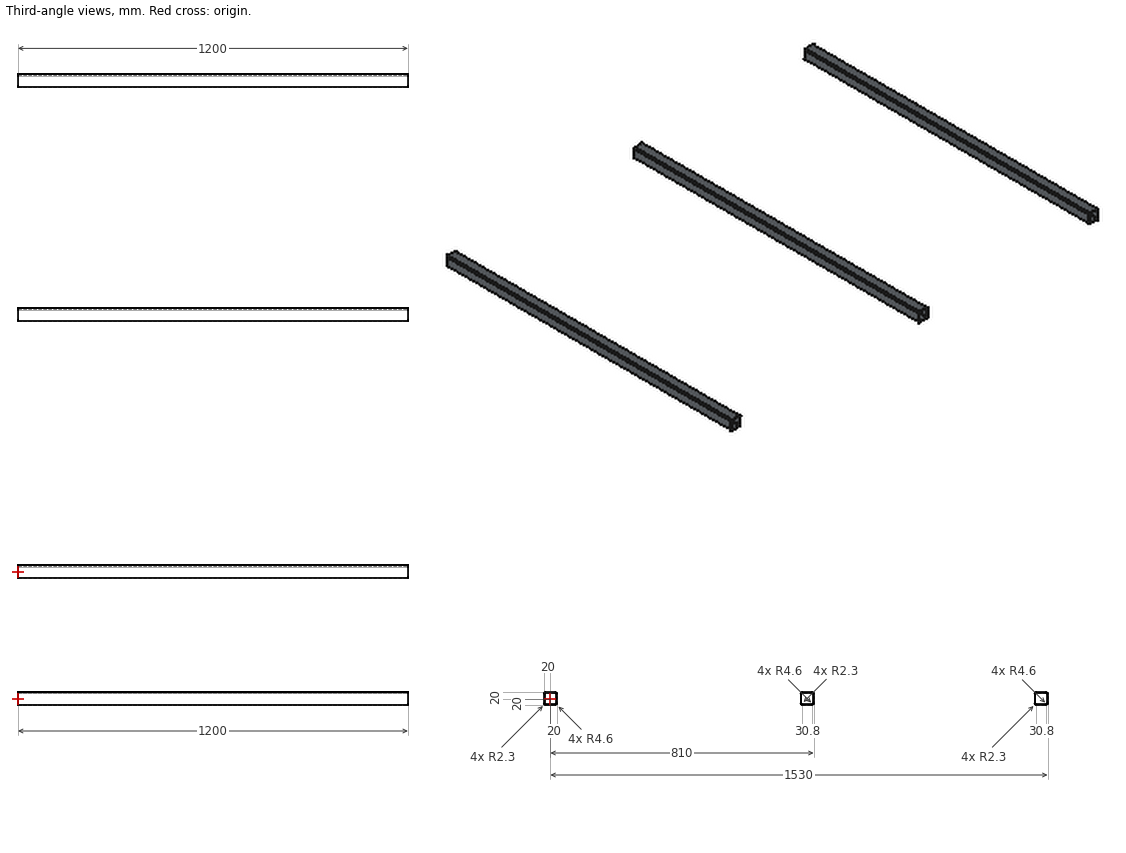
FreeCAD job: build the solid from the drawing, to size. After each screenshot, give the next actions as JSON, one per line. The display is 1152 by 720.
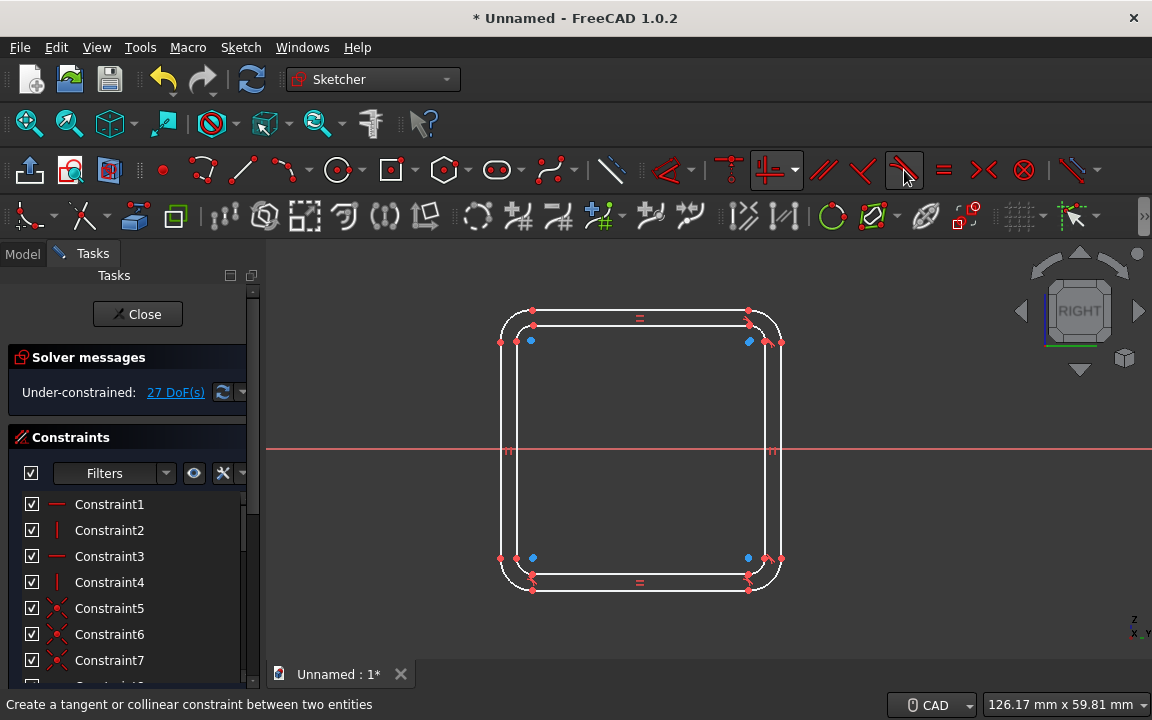
{"action": "left_click", "coordinate": [684, 310]}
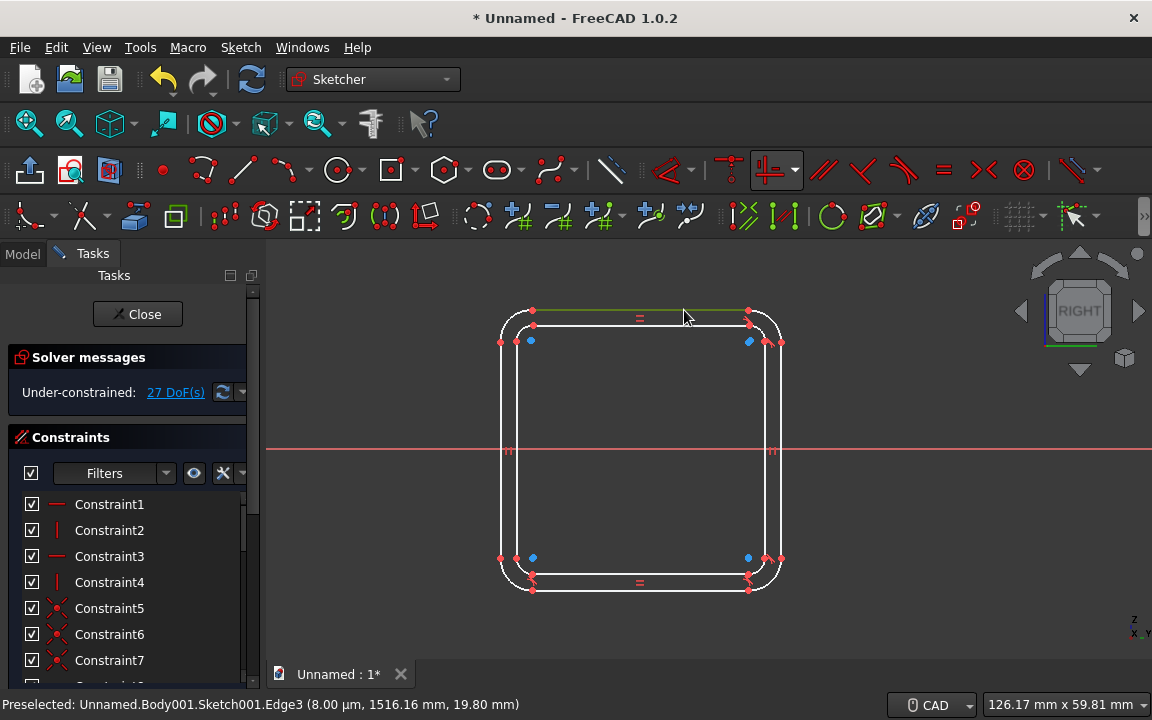
{"action": "left_click", "coordinate": [518, 313]}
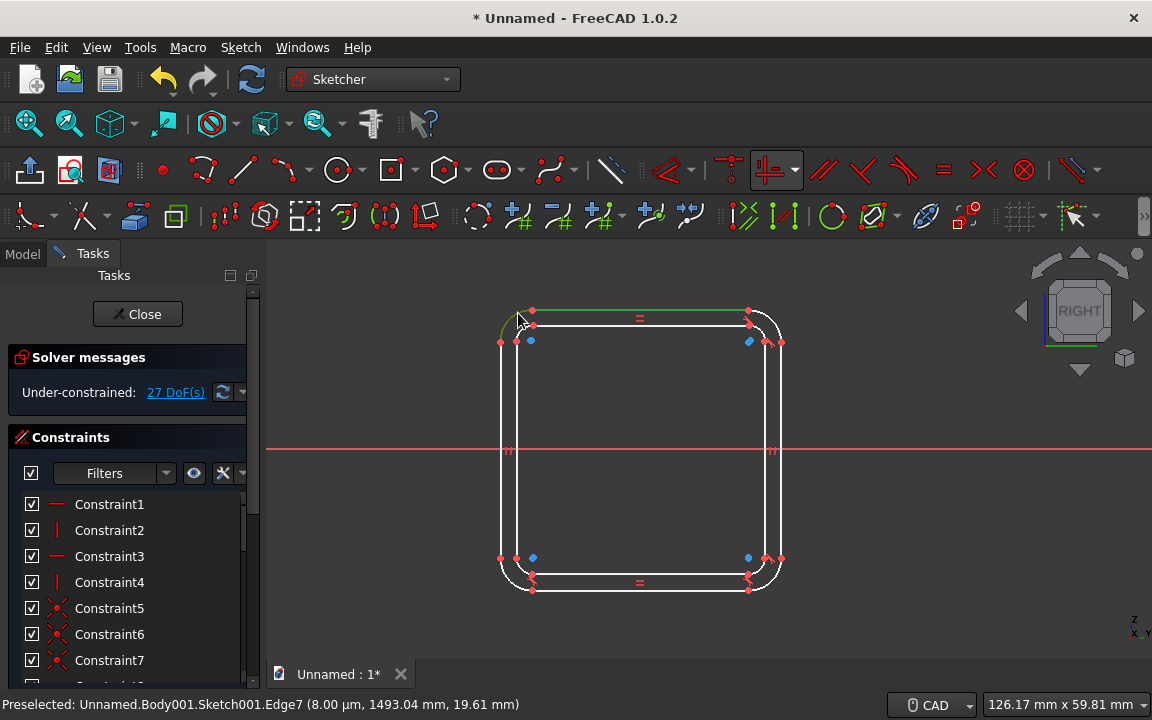
{"action": "left_click", "coordinate": [904, 170]}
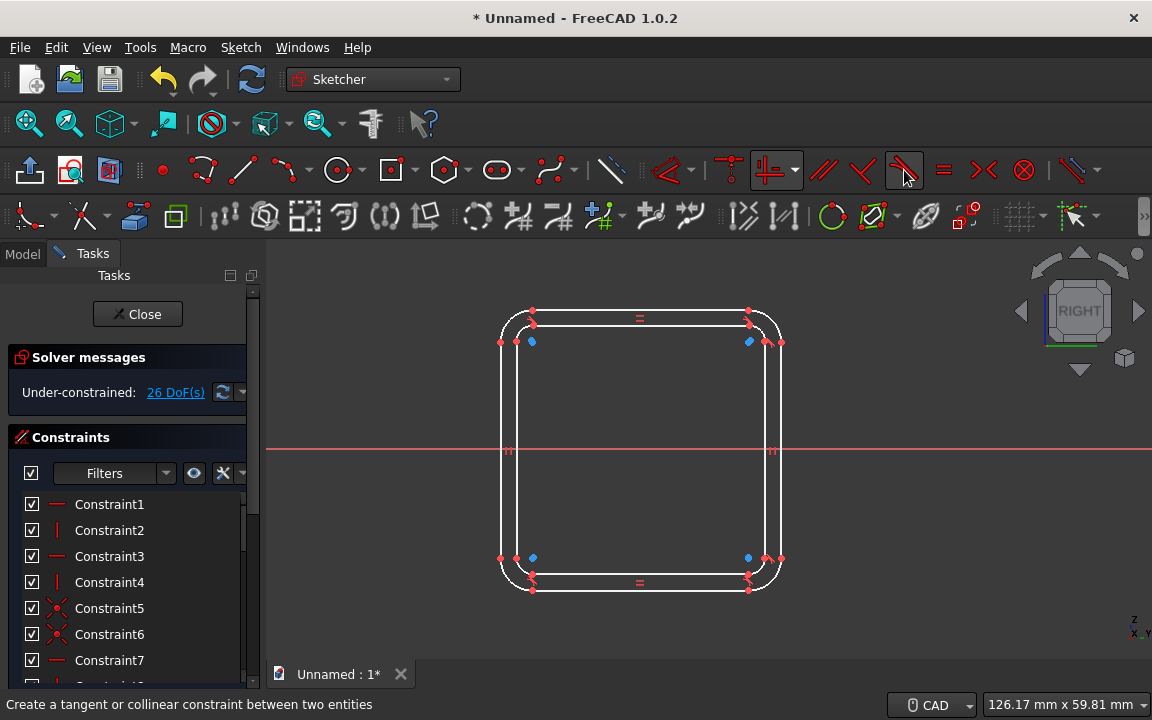
{"action": "left_click", "coordinate": [501, 407]}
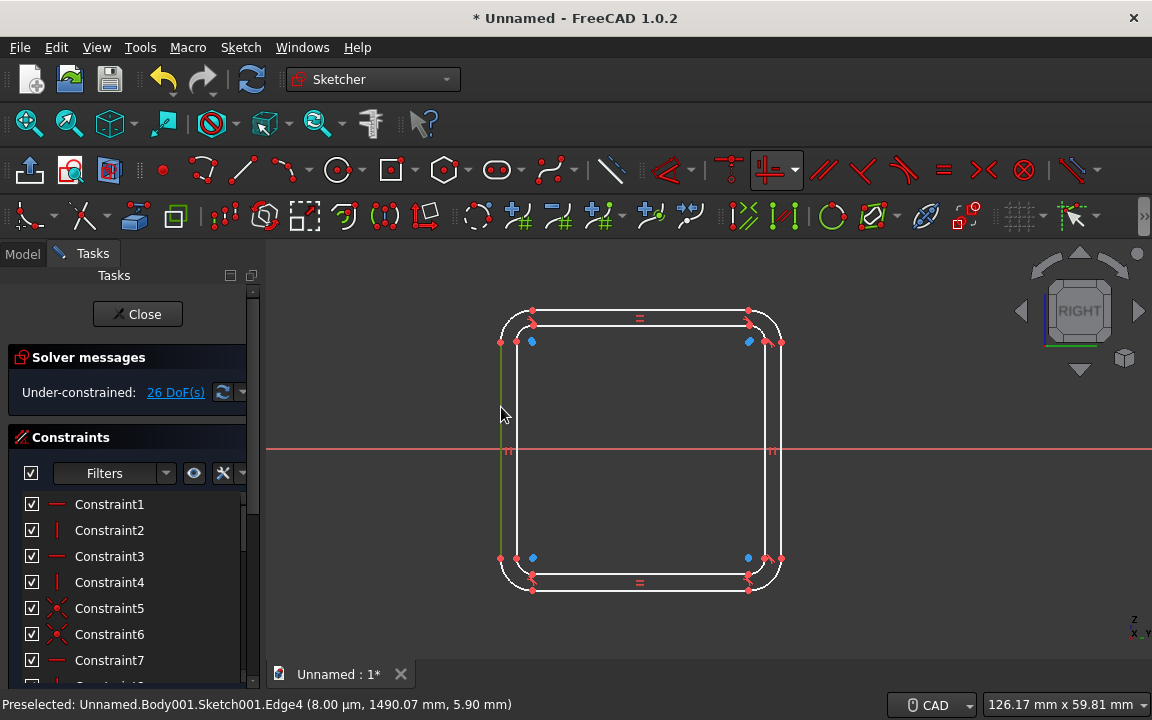
{"action": "left_click", "coordinate": [518, 314]}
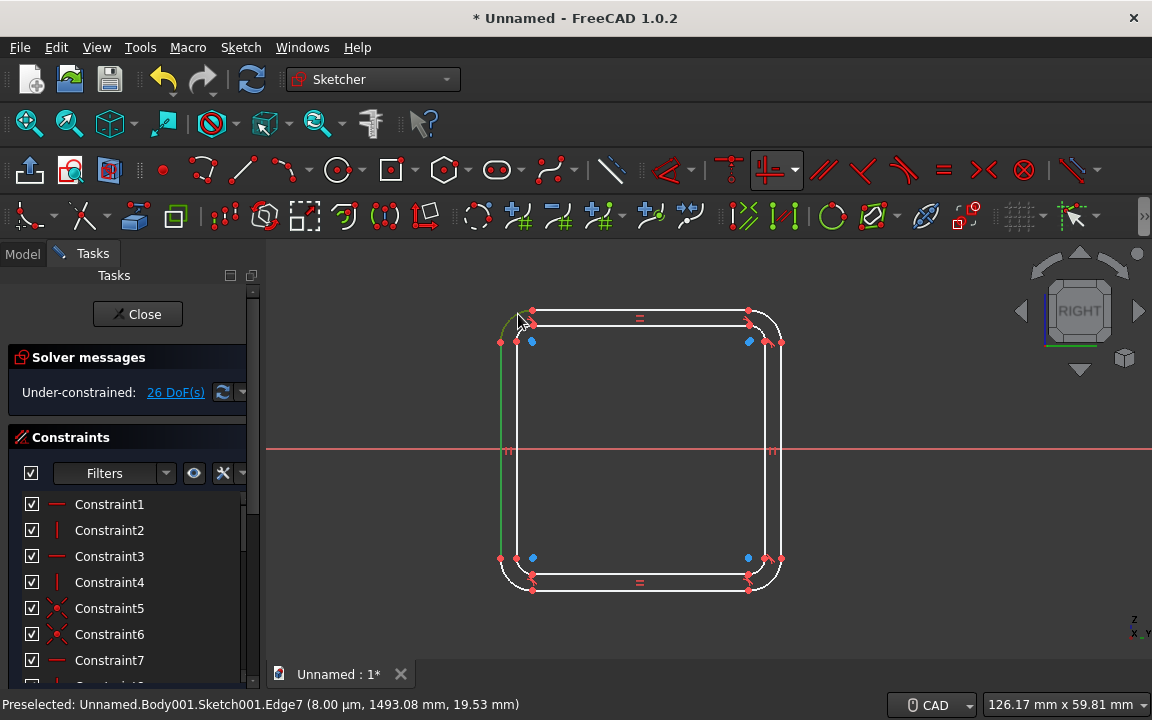
{"action": "key", "text": "t"}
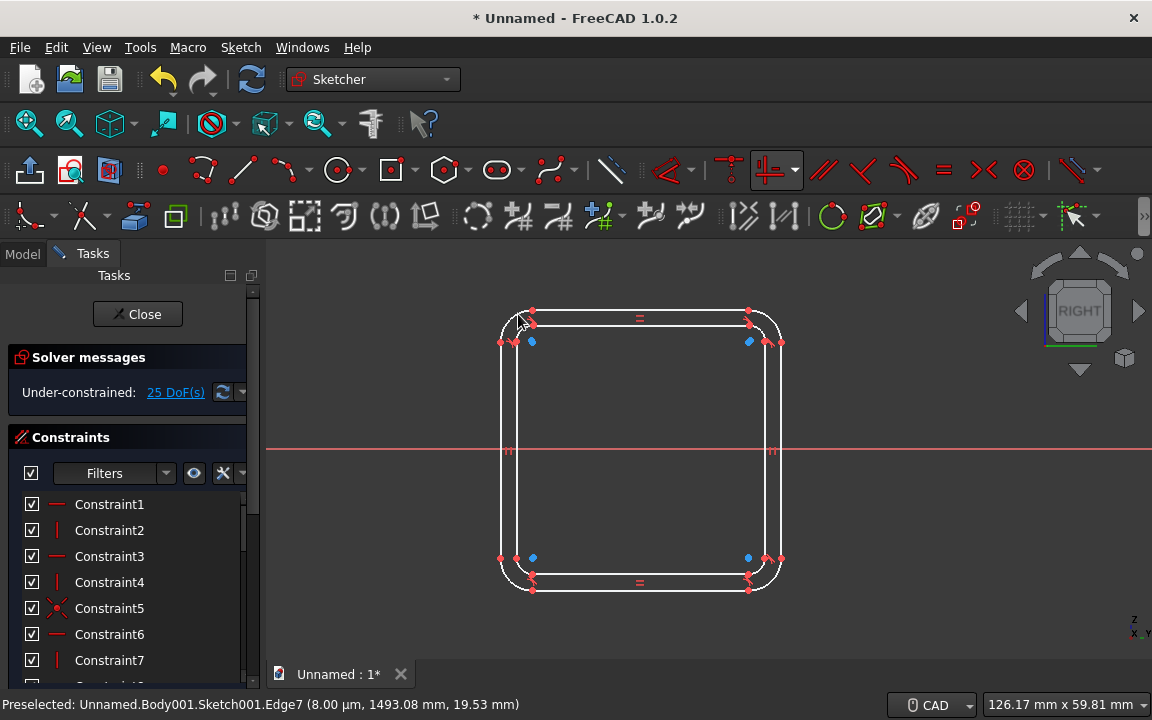
{"action": "left_click", "coordinate": [501, 407]}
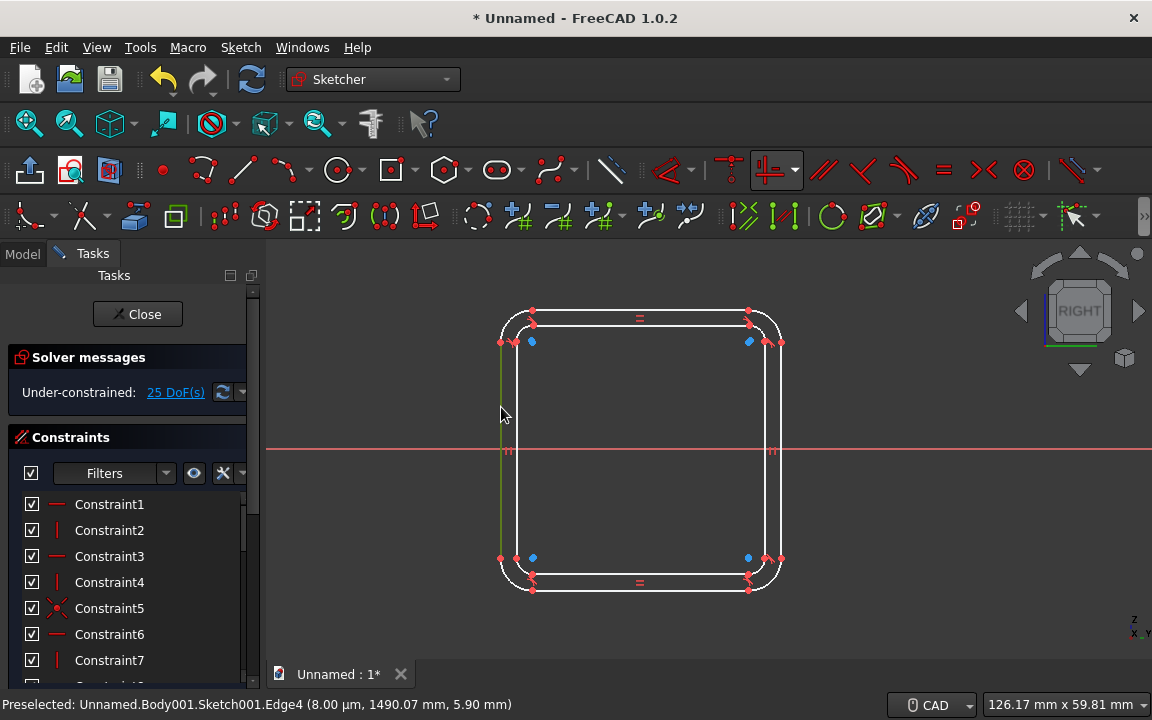
{"action": "left_click", "coordinate": [504, 573]}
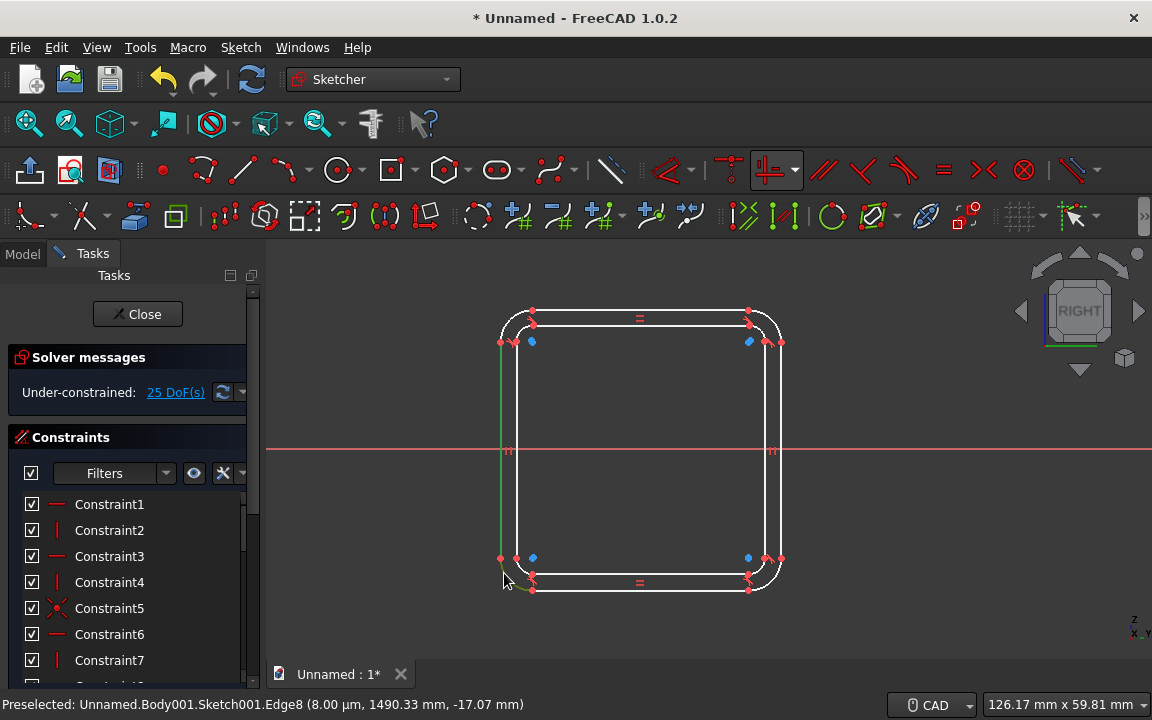
{"action": "key", "text": "t"}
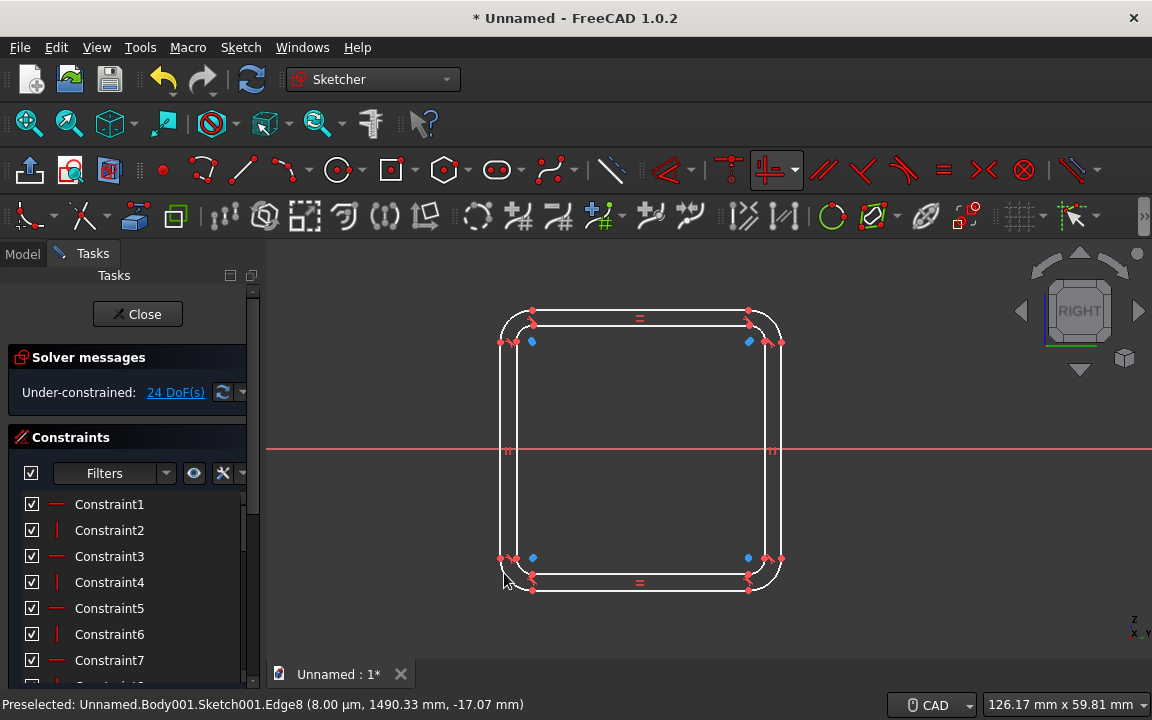
{"action": "left_click", "coordinate": [684, 574]}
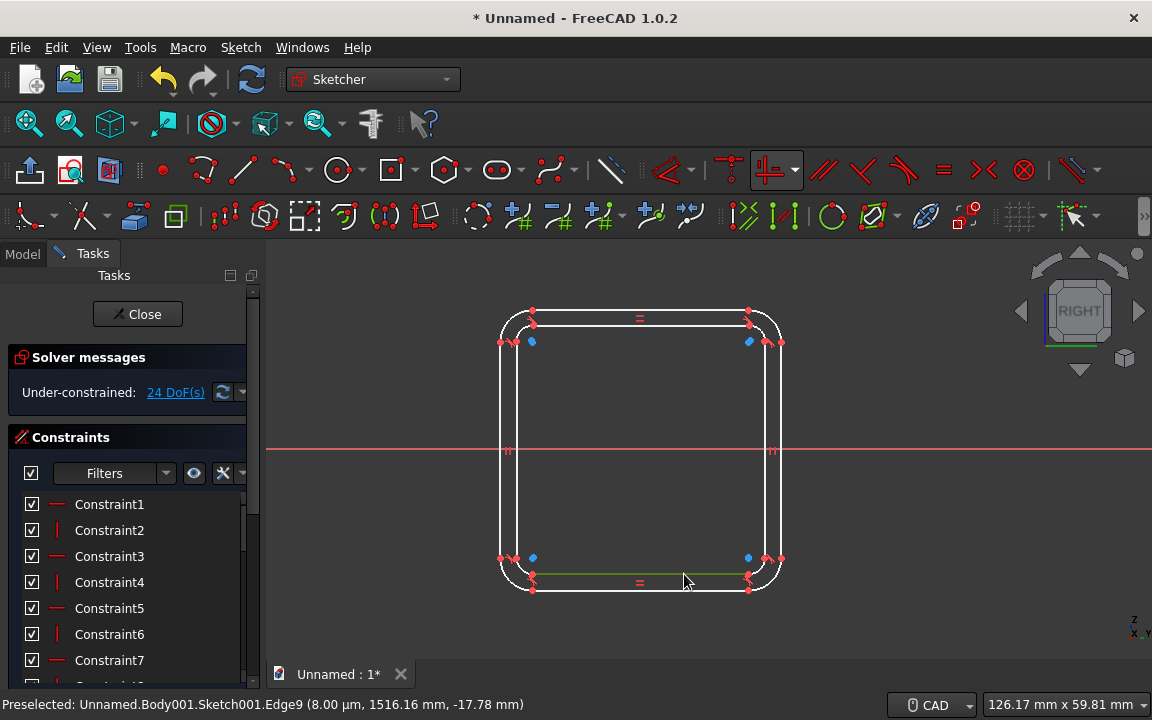
{"action": "left_click", "coordinate": [522, 569]}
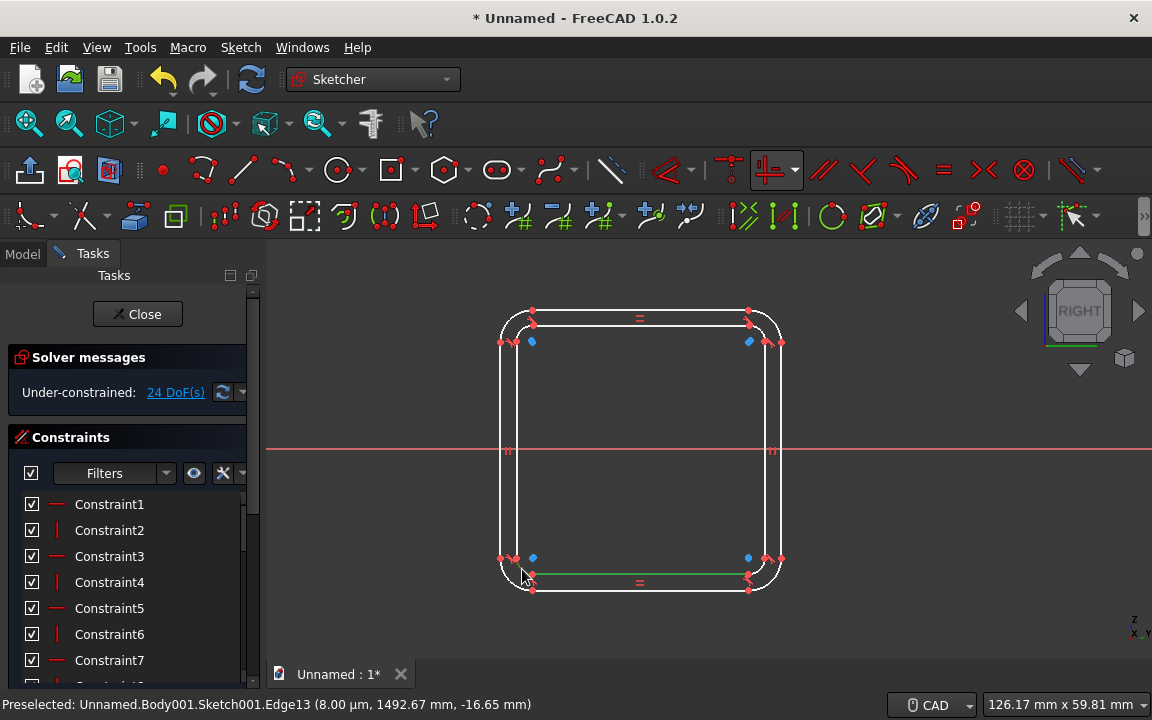
{"action": "key", "text": "t"}